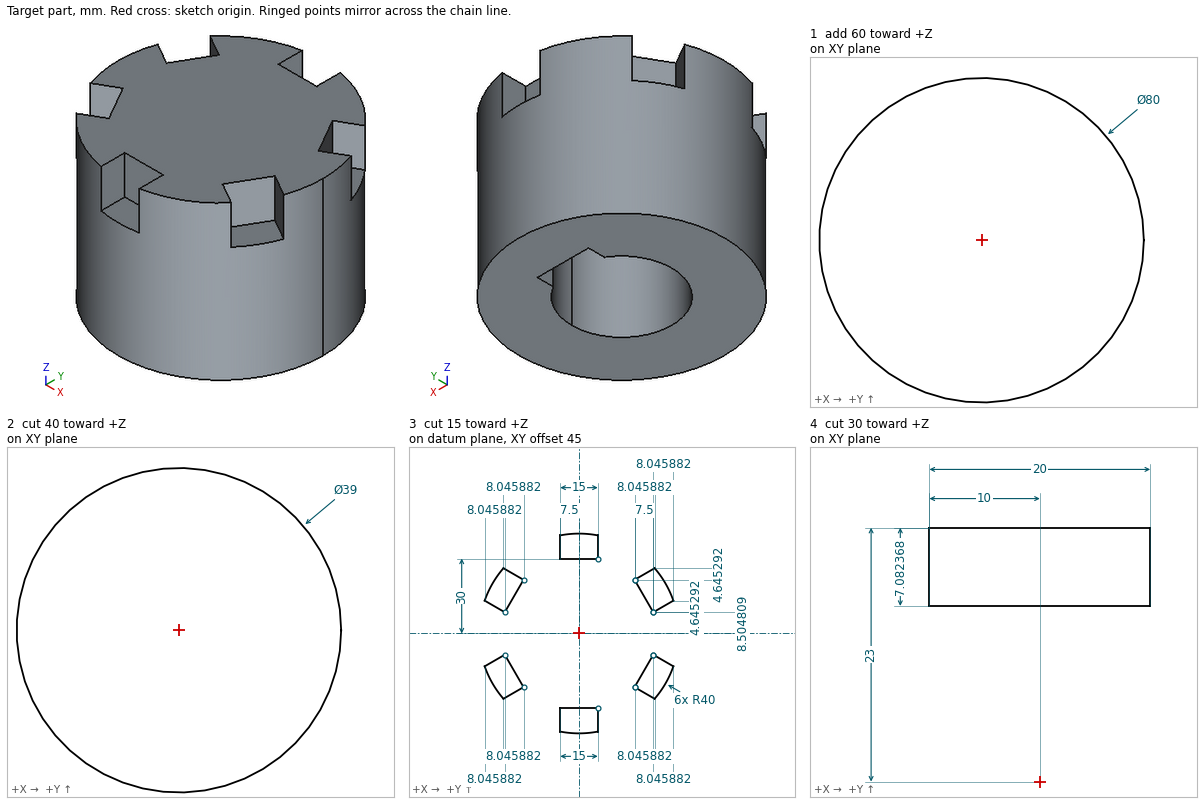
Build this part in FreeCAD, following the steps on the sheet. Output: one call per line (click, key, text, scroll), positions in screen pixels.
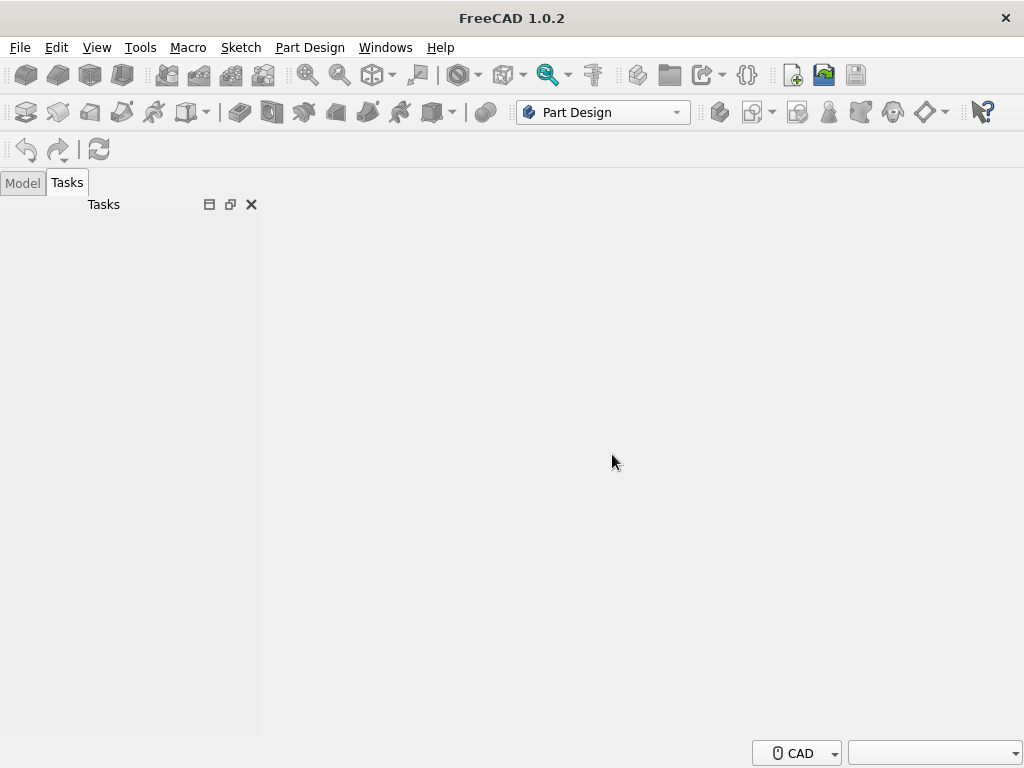
click(792, 76)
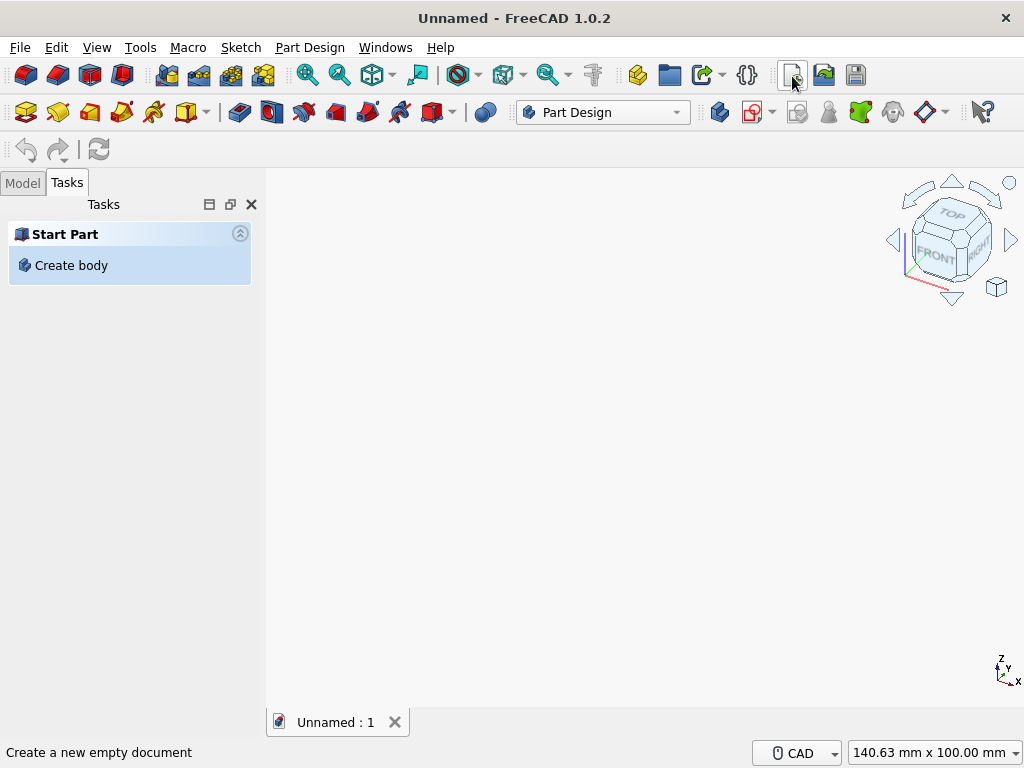
click(752, 112)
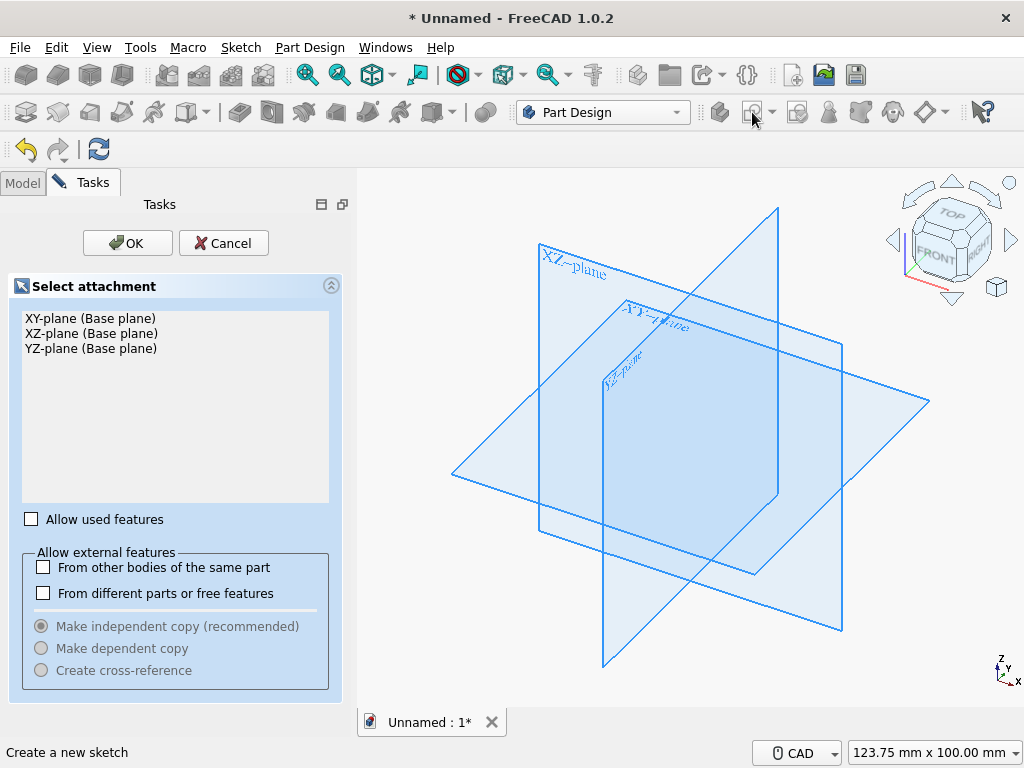
click(82, 318)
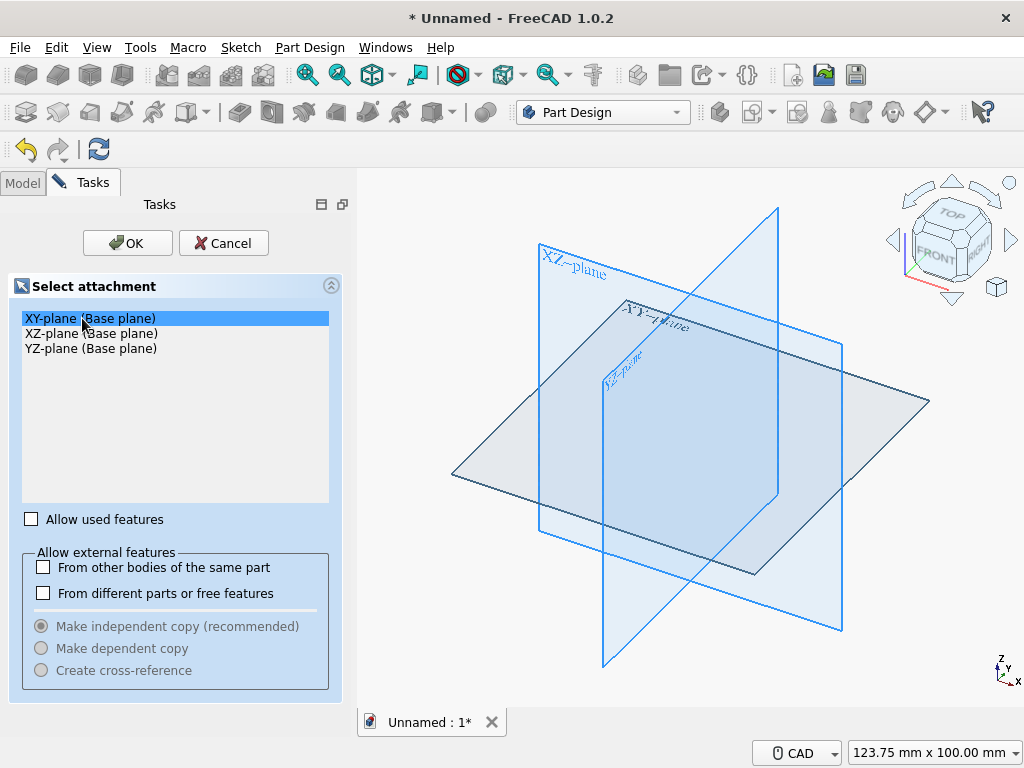
click(128, 243)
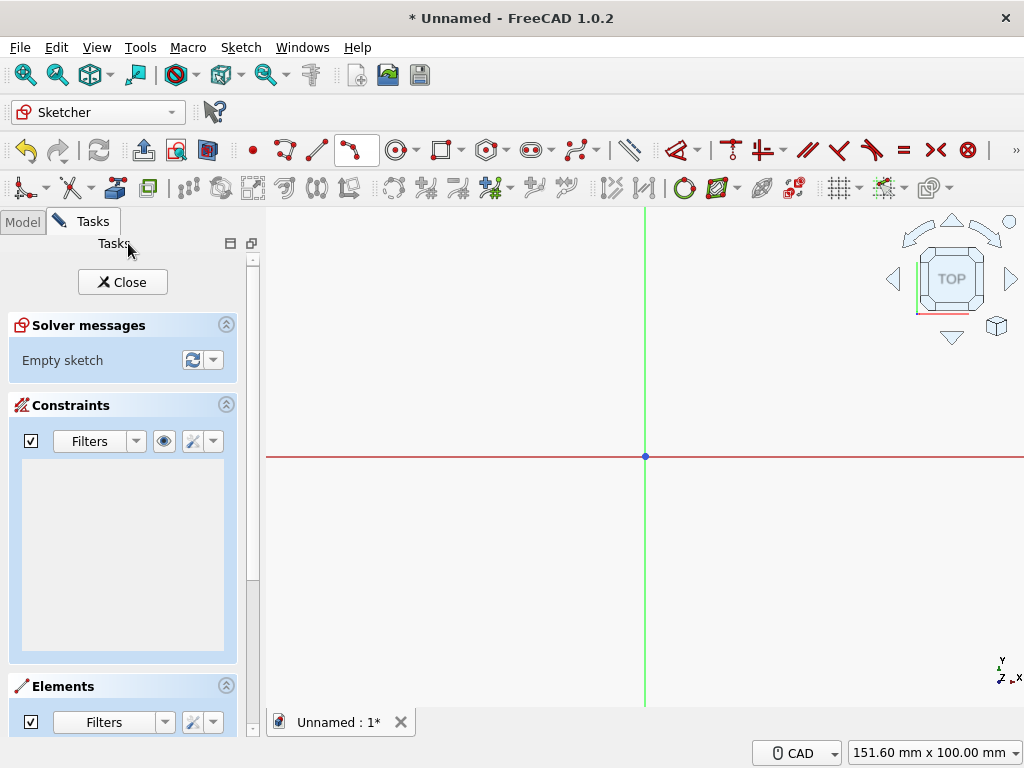
scroll(294, 457, down, 1)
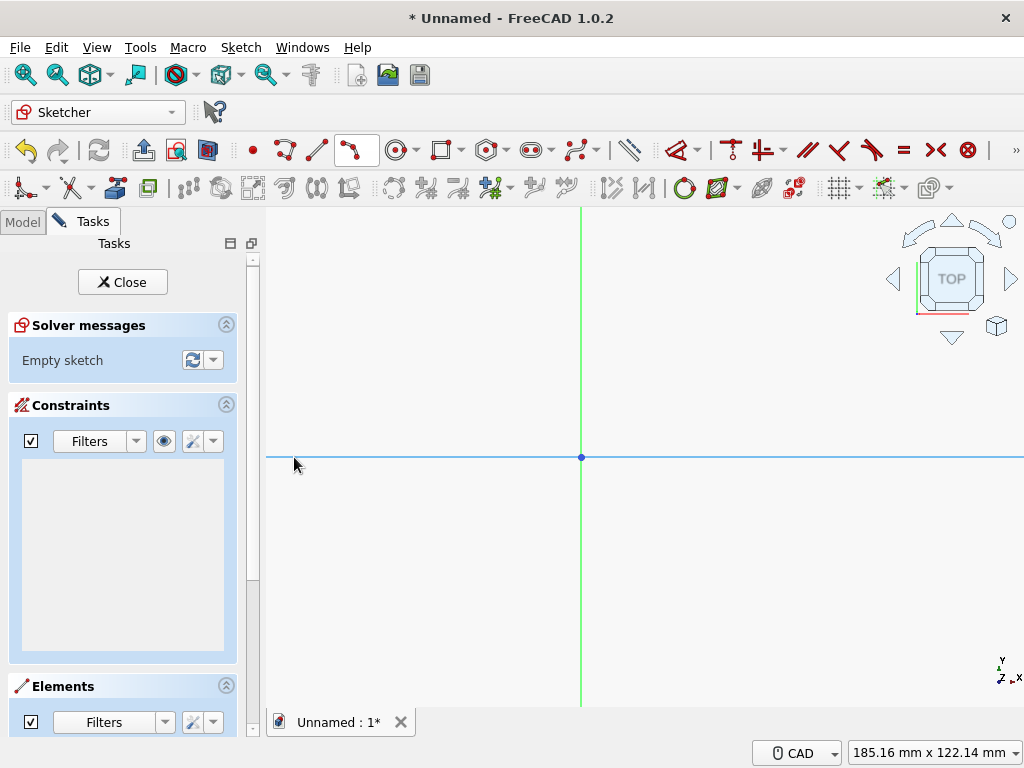
key(g)
key(c)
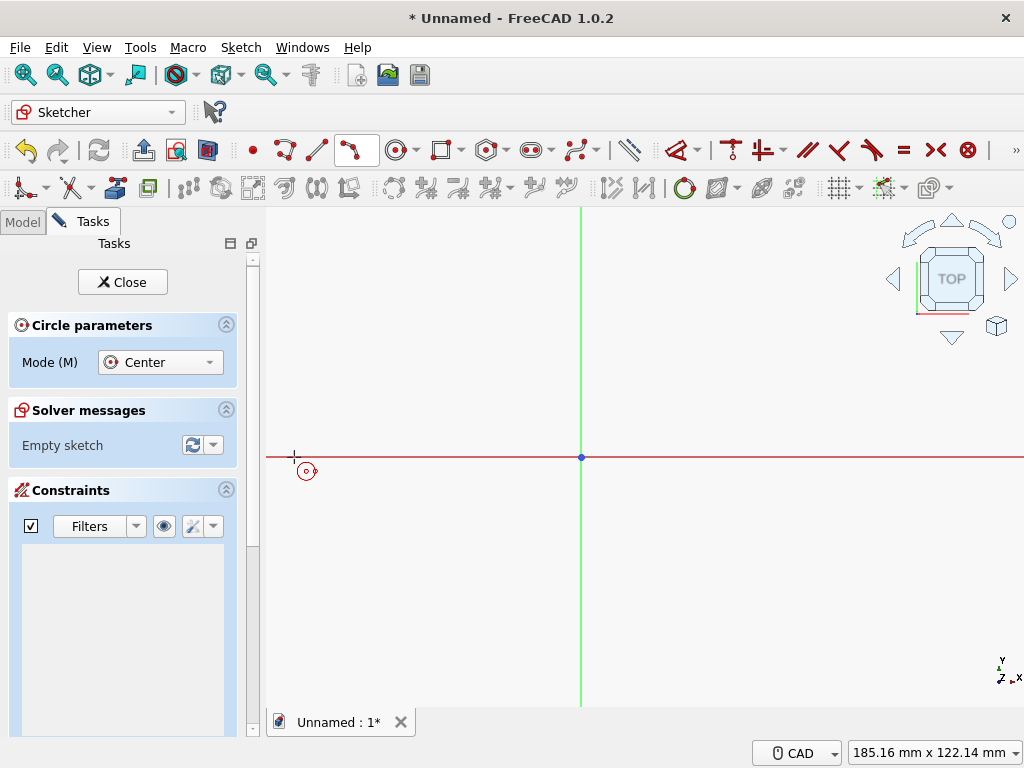
click(581, 457)
click(697, 341)
key(Escape)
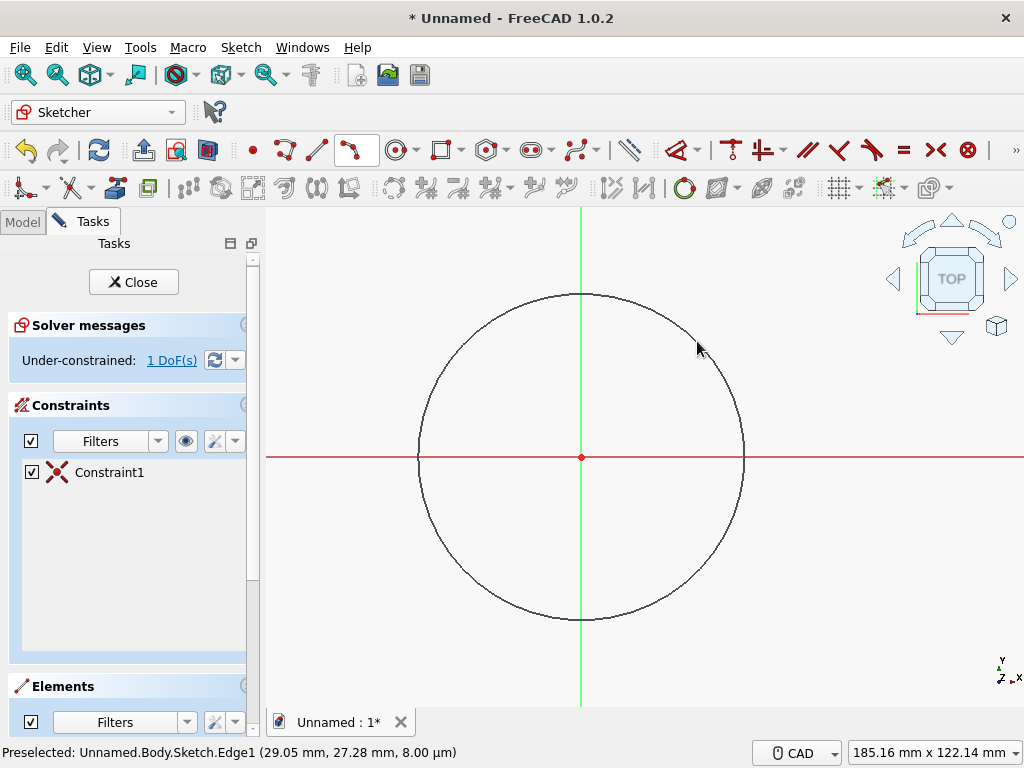
click(676, 150)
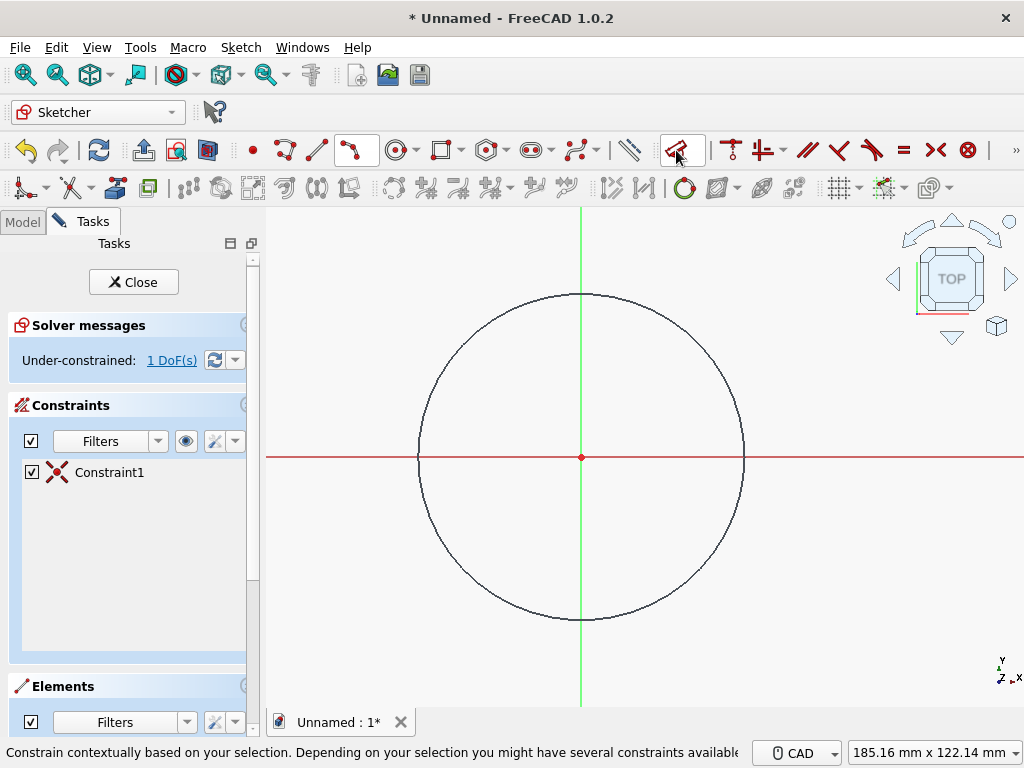
click(696, 341)
click(718, 318)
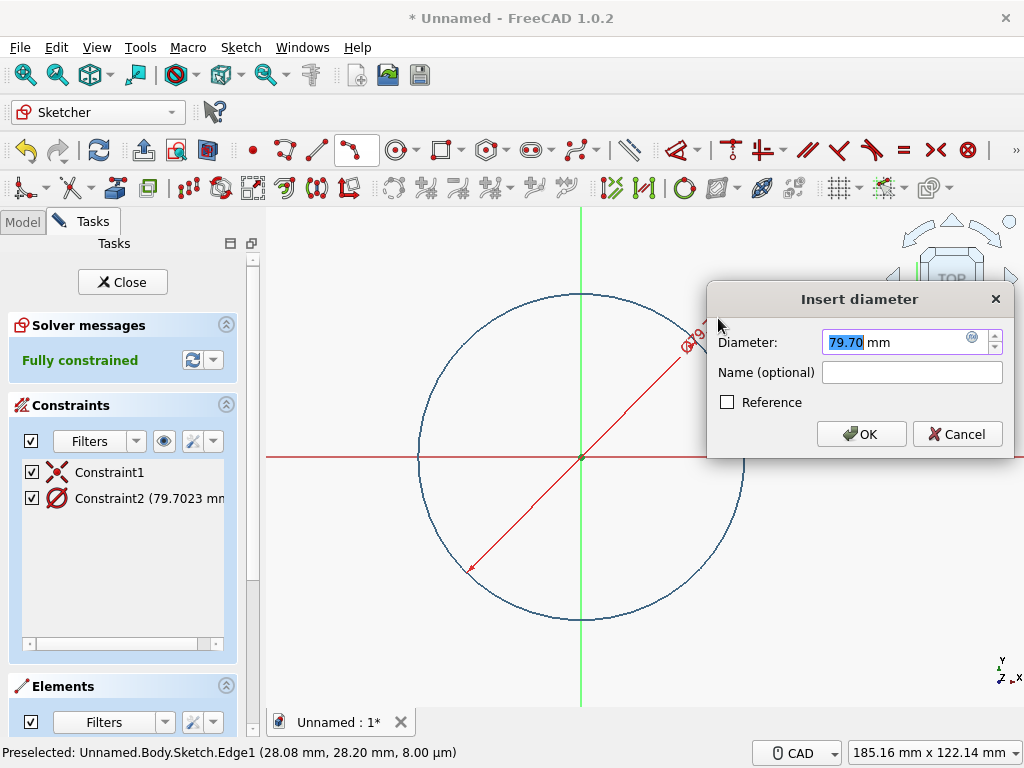
text(80)
key(Return)
key(Escape)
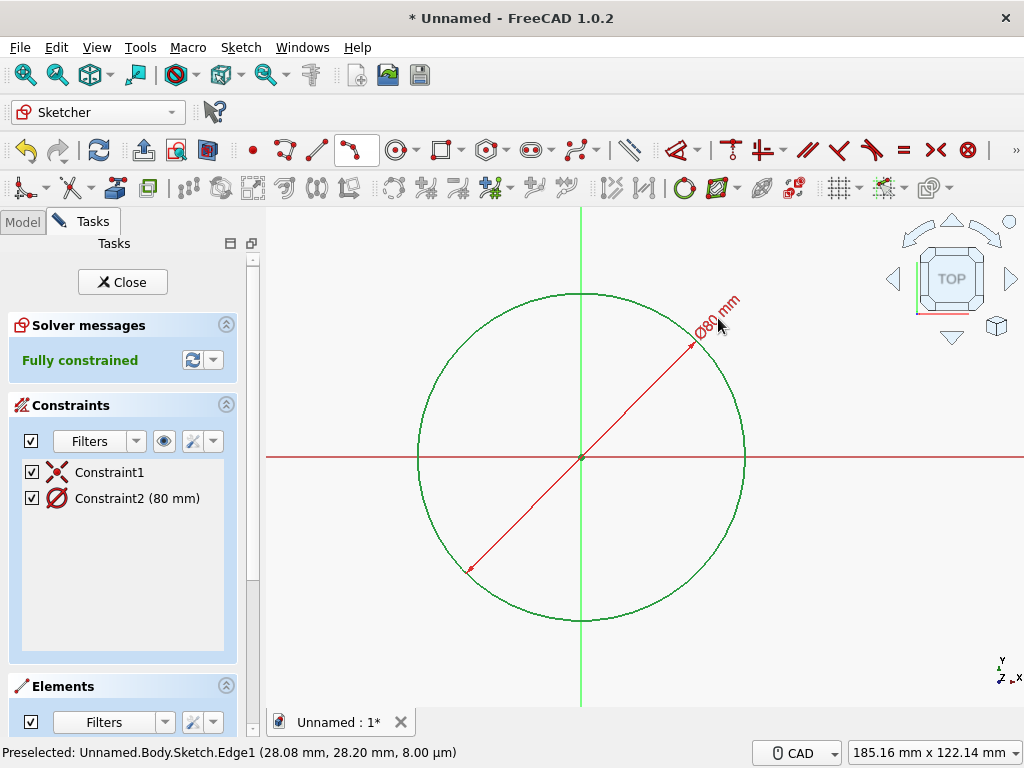
click(123, 282)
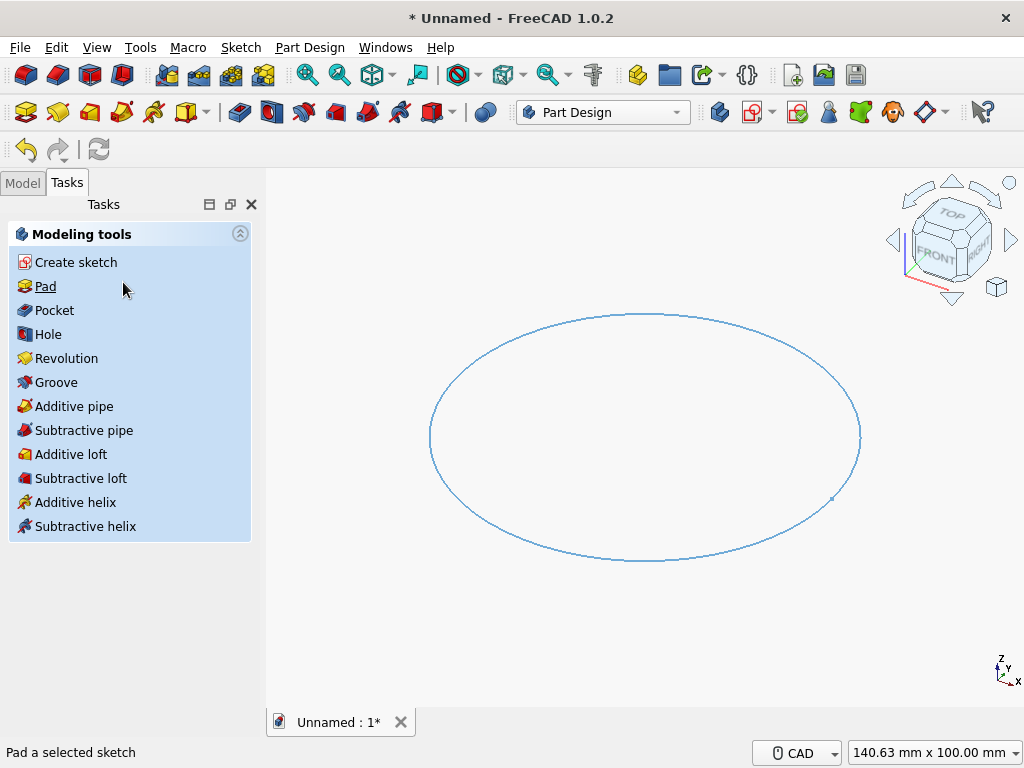
click(26, 112)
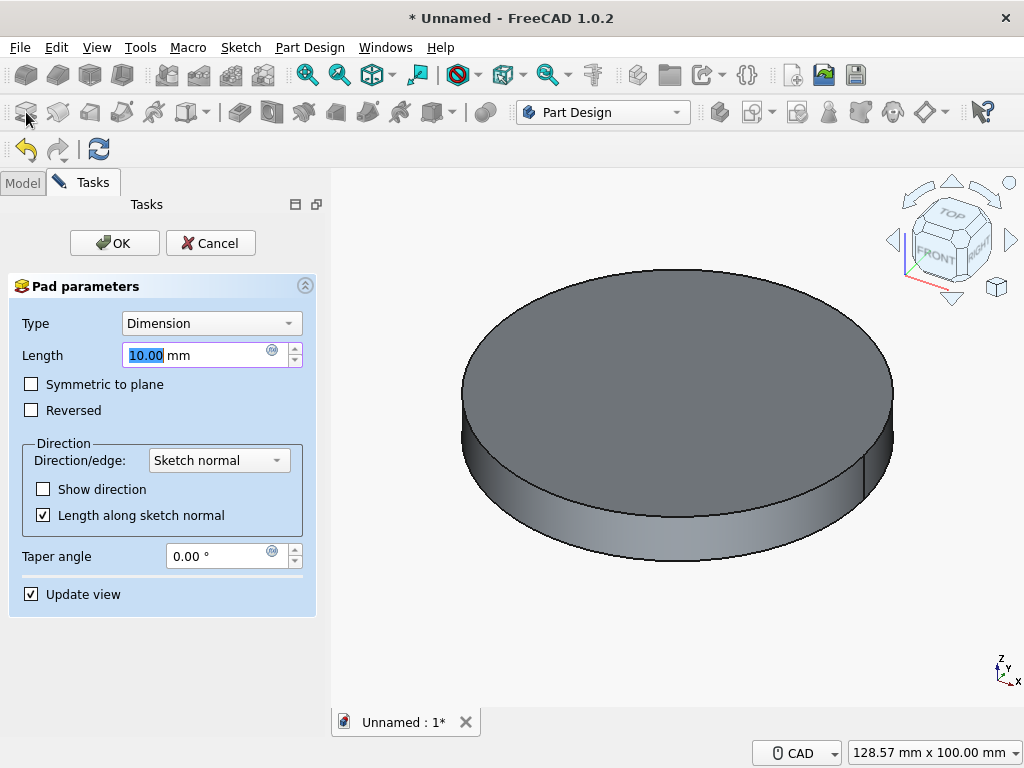
text(60)
key(Tab)